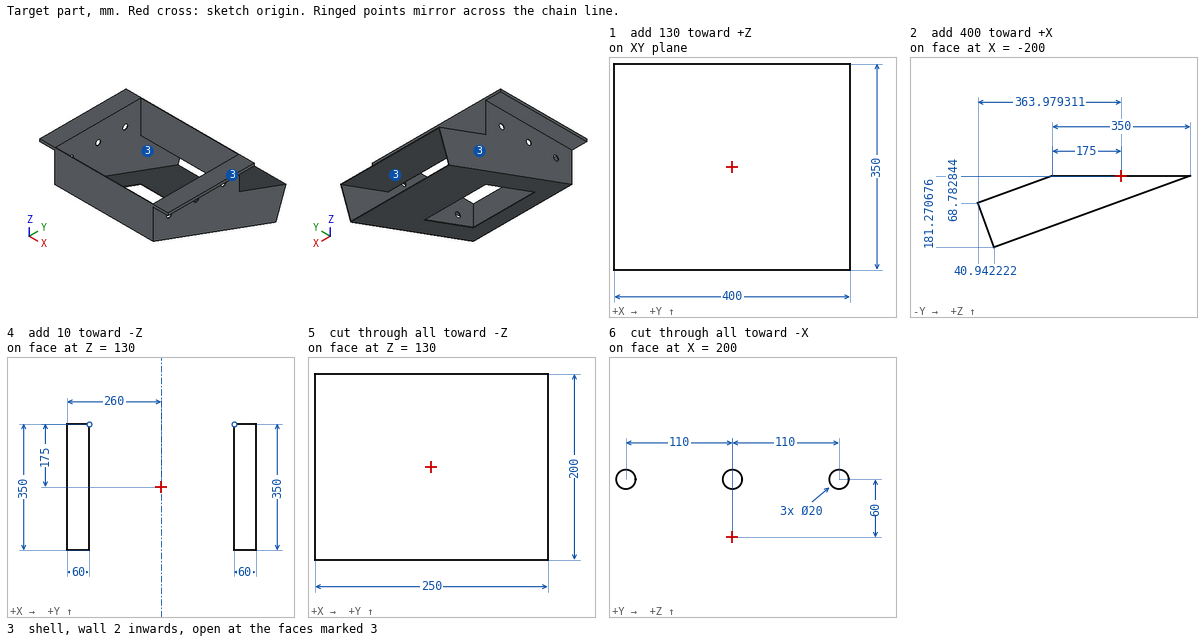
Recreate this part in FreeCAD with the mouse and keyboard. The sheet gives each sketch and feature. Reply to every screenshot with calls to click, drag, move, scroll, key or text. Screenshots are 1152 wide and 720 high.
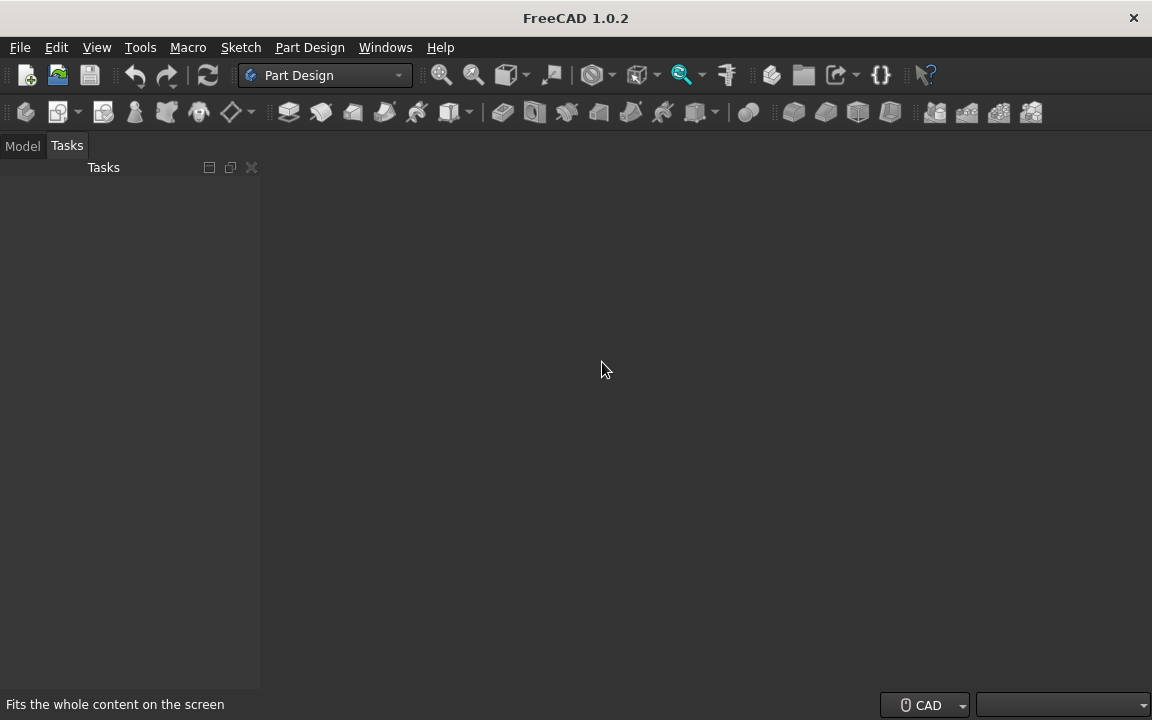
click(26, 76)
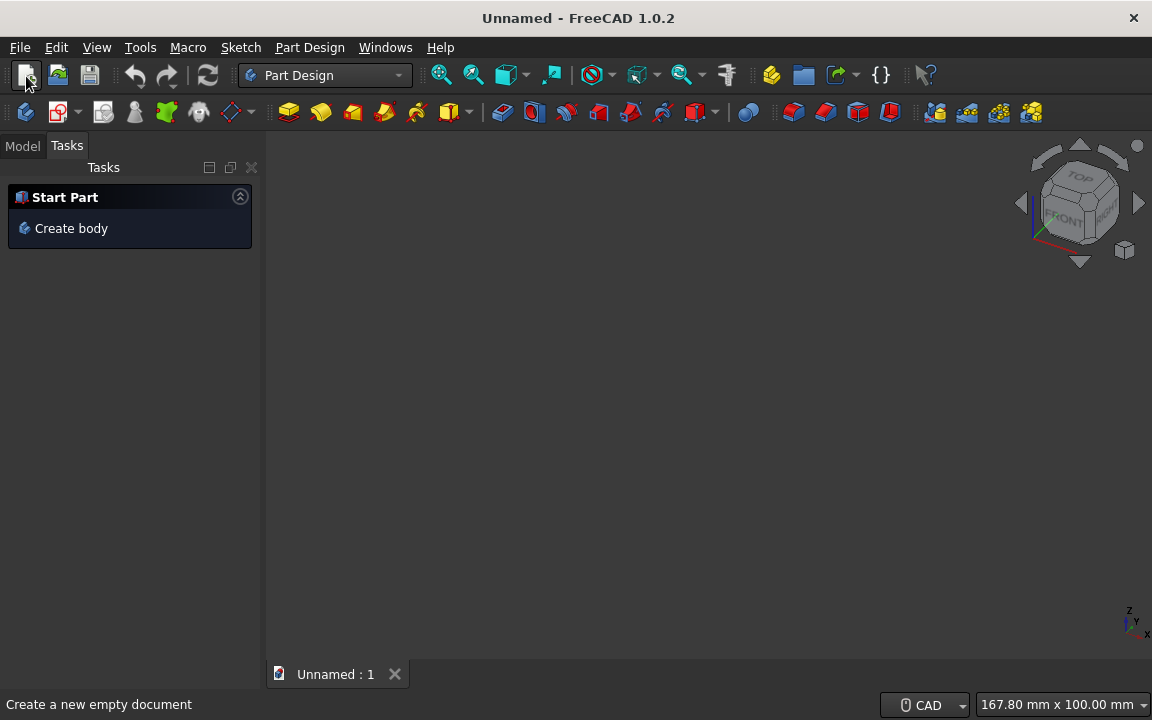
click(58, 112)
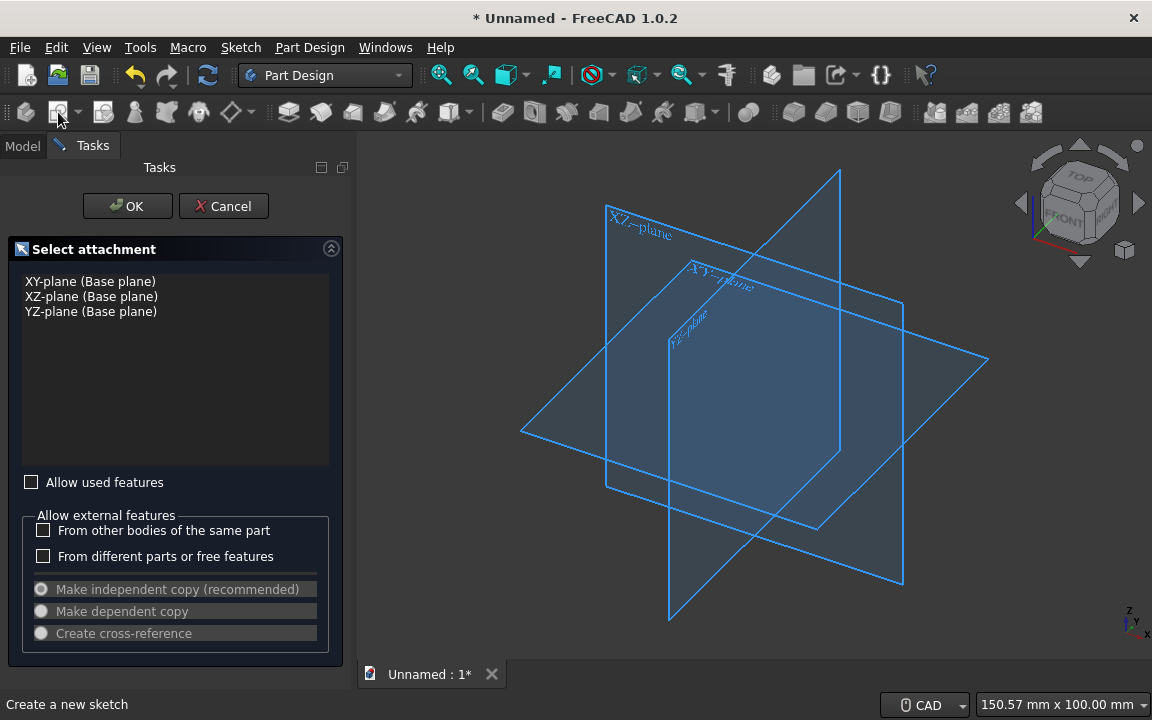
click(82, 282)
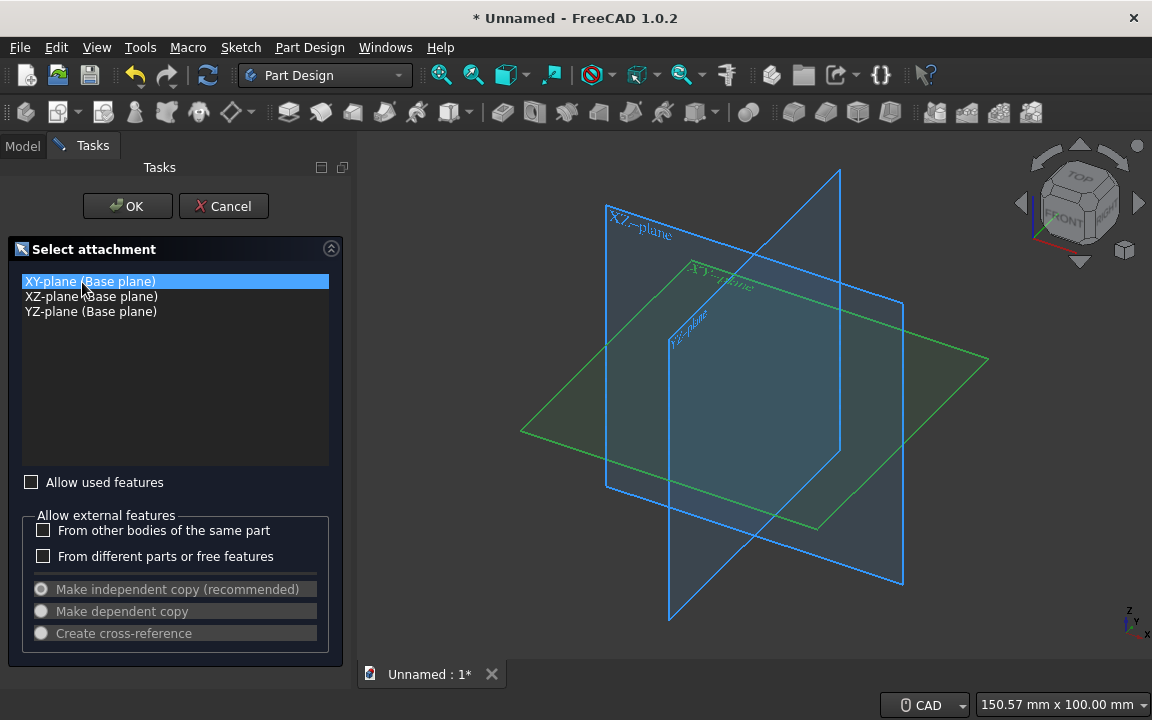
click(128, 206)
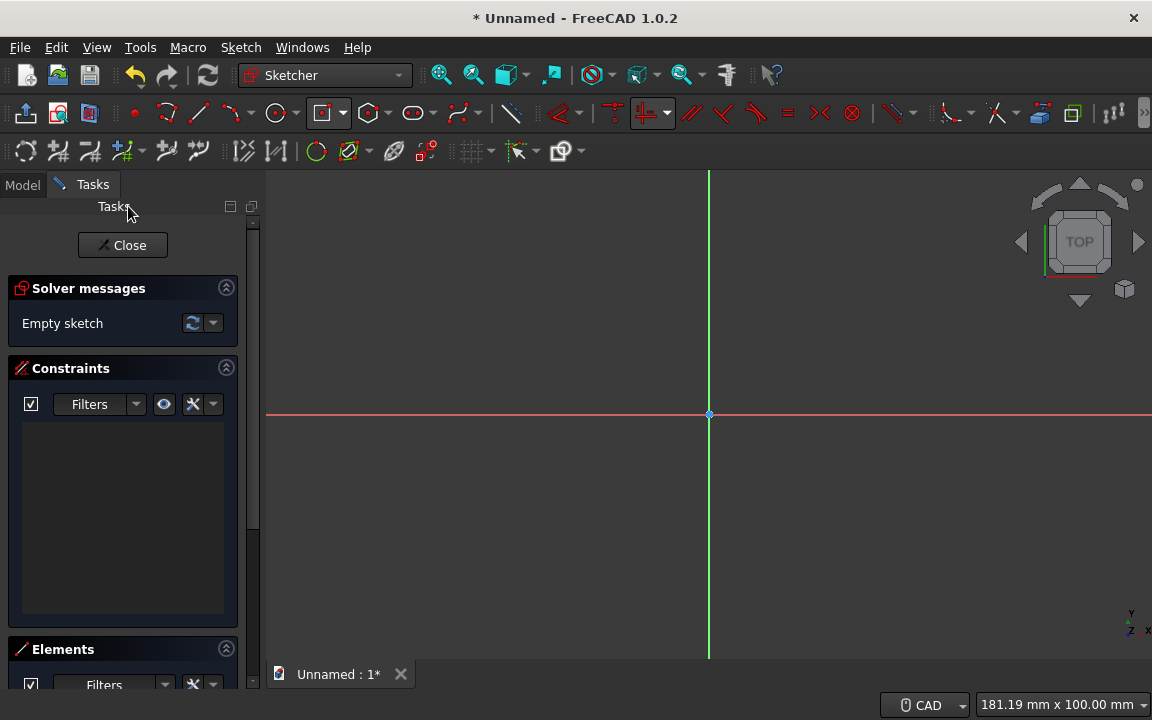
scroll(627, 415, down, 9)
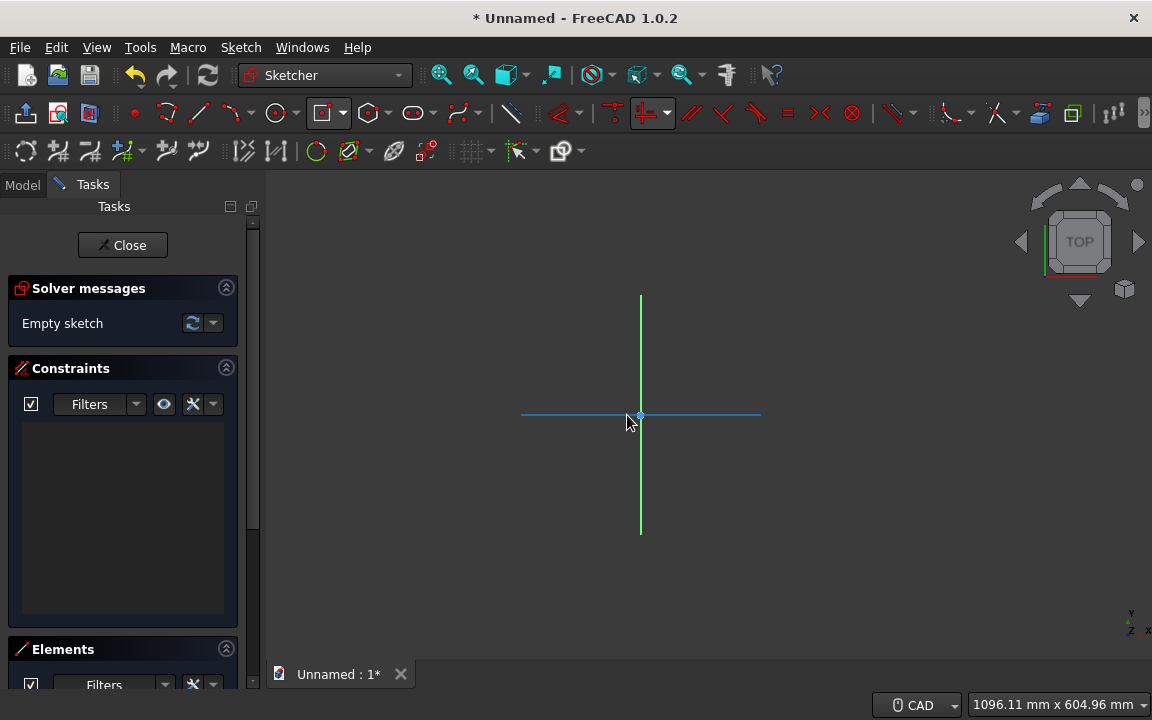
click(322, 114)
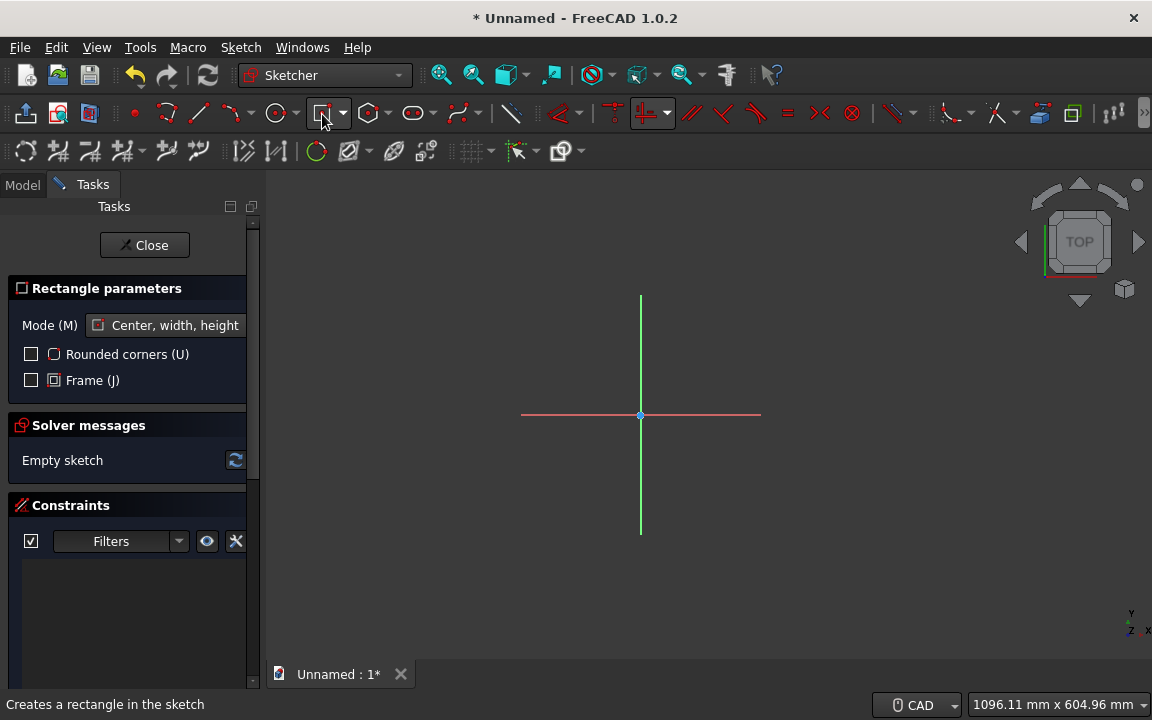
click(641, 415)
move(803, 274)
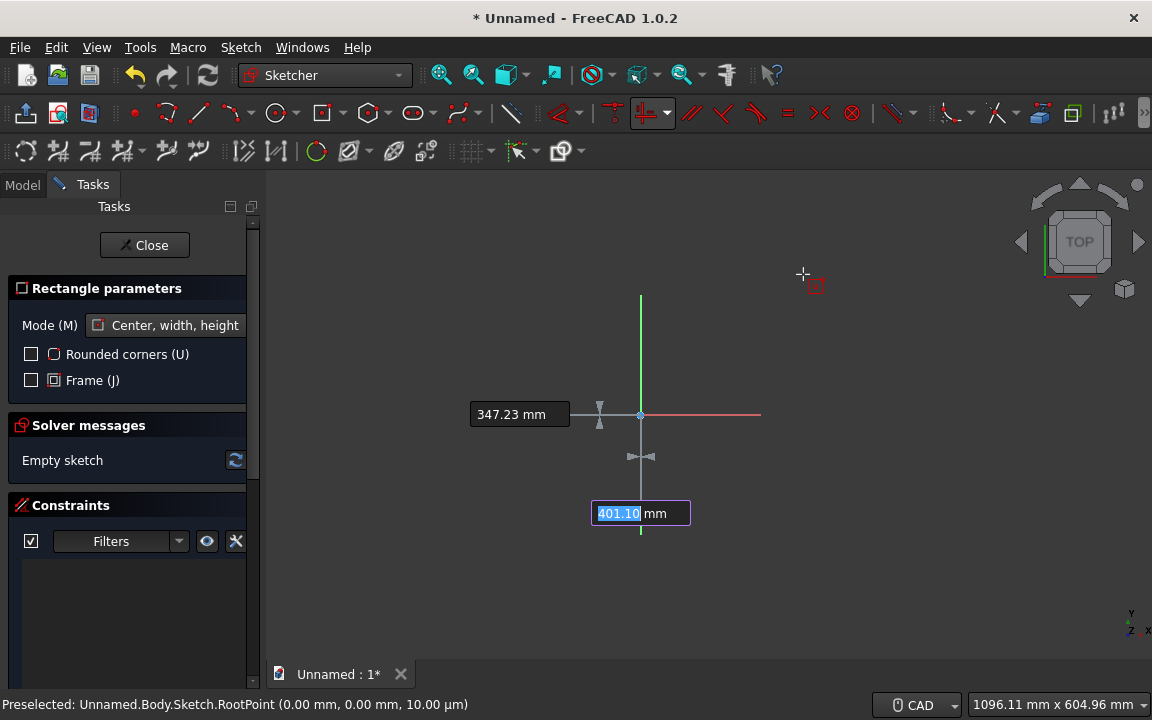
text(400)
key(Tab)
text(350)
key(Return)
key(Escape)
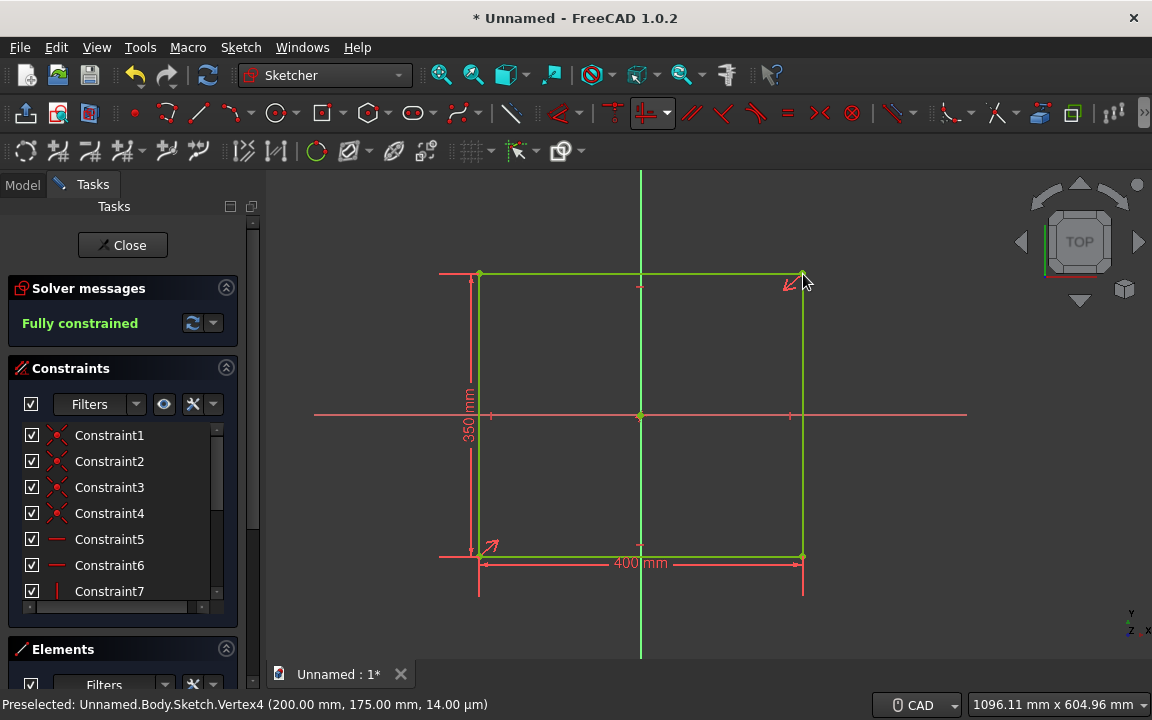
click(123, 245)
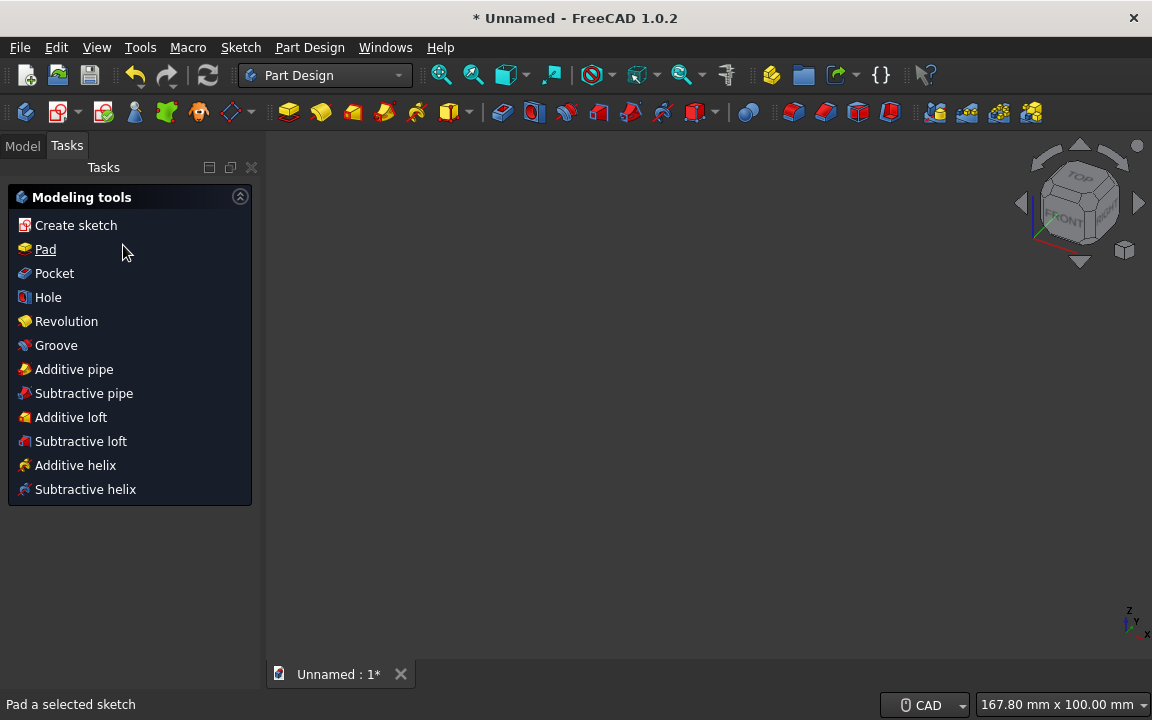
click(290, 112)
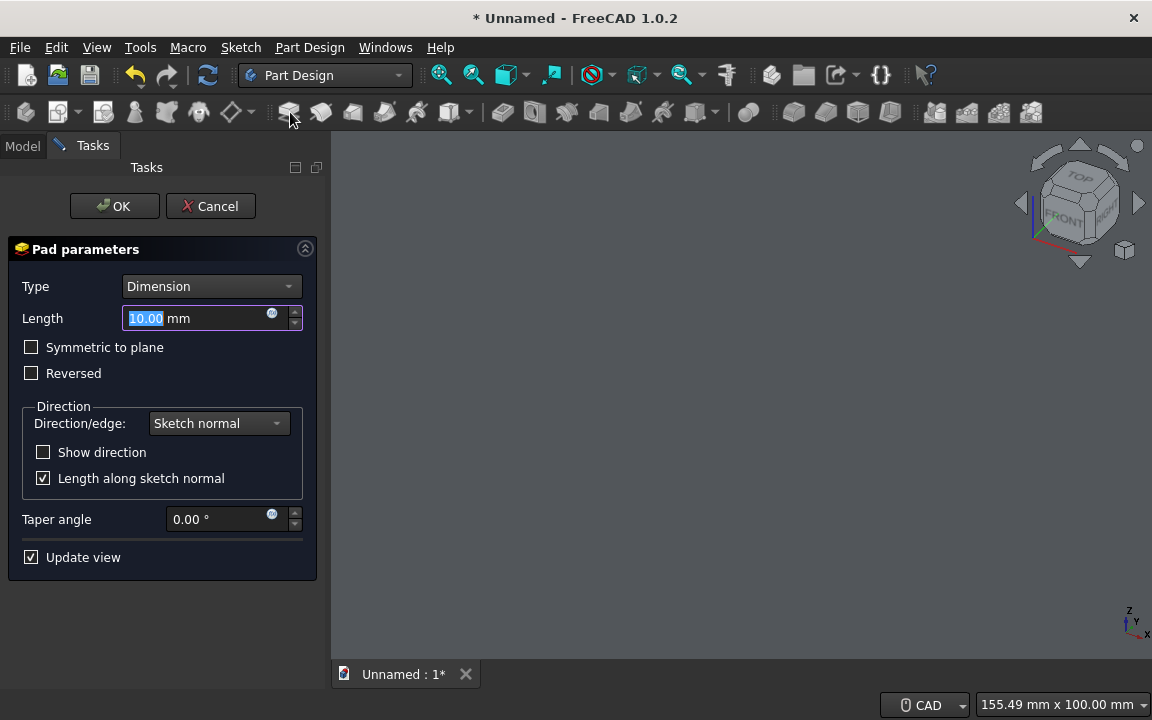
text(130)
key(Tab)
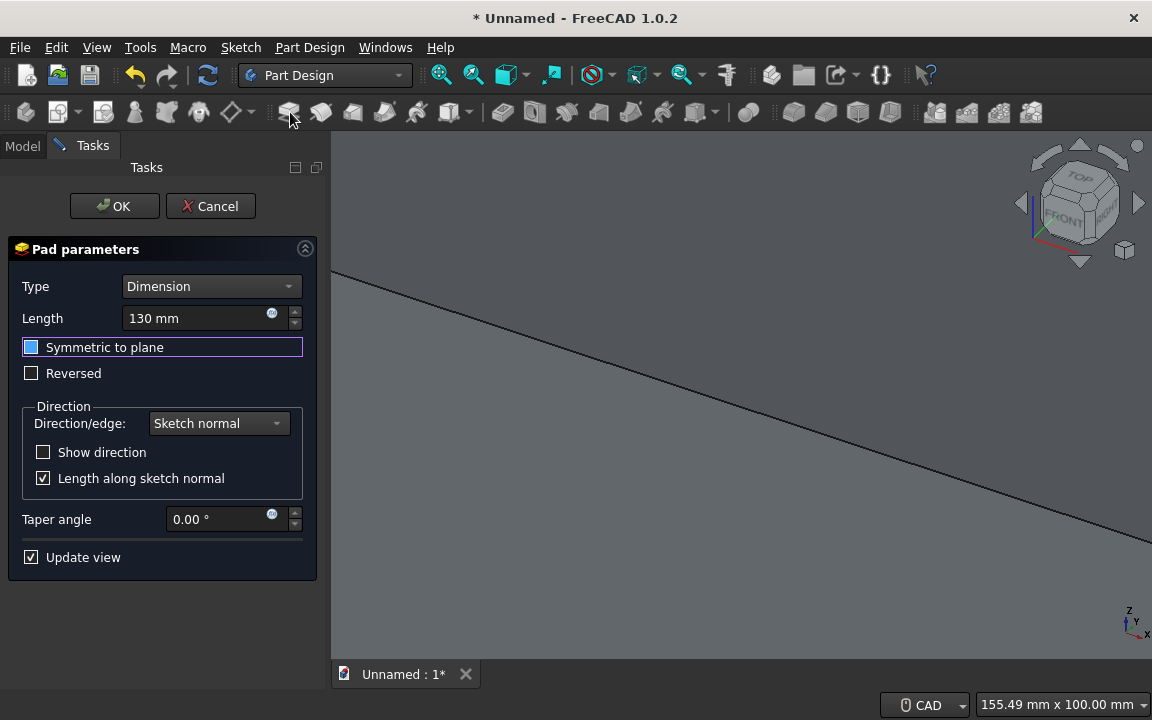
click(115, 206)